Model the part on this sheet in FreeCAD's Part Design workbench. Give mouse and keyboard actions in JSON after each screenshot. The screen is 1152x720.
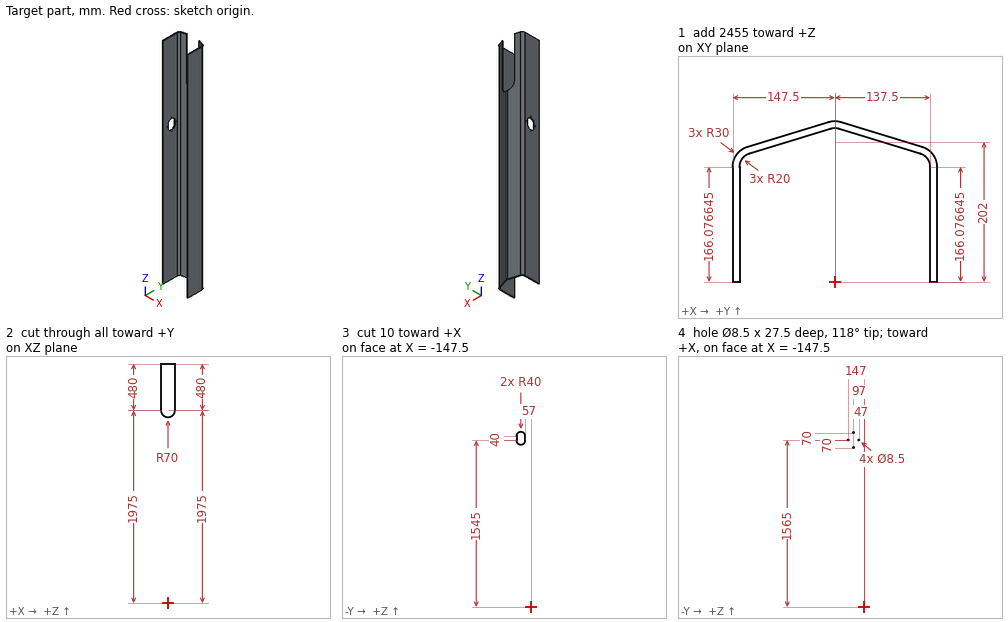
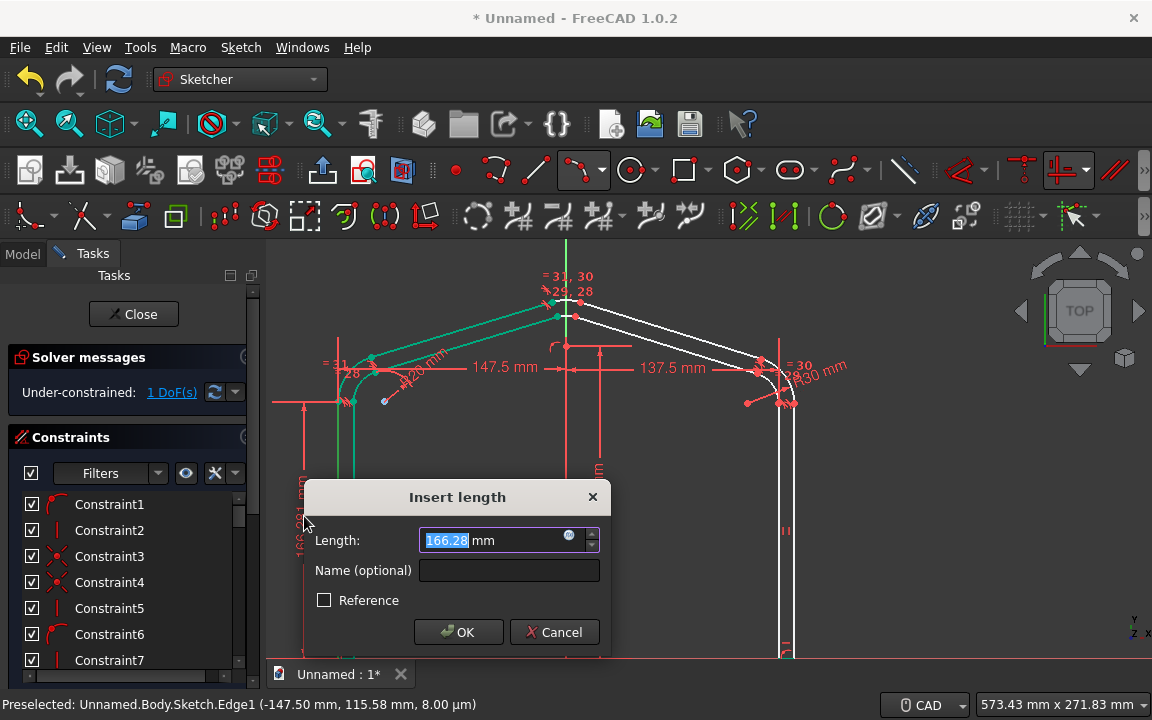
{"action": "type", "text": "166.076645"}
{"action": "key", "text": "Return"}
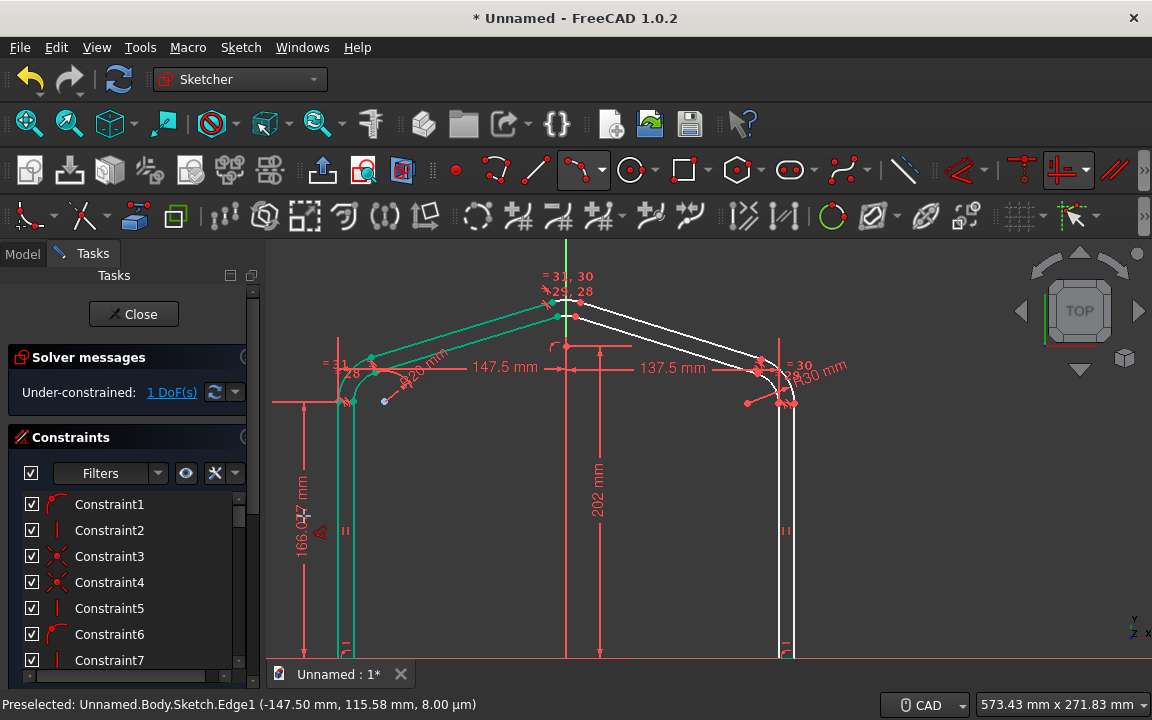
{"action": "left_click", "coordinate": [779, 480]}
{"action": "left_click", "coordinate": [813, 517]}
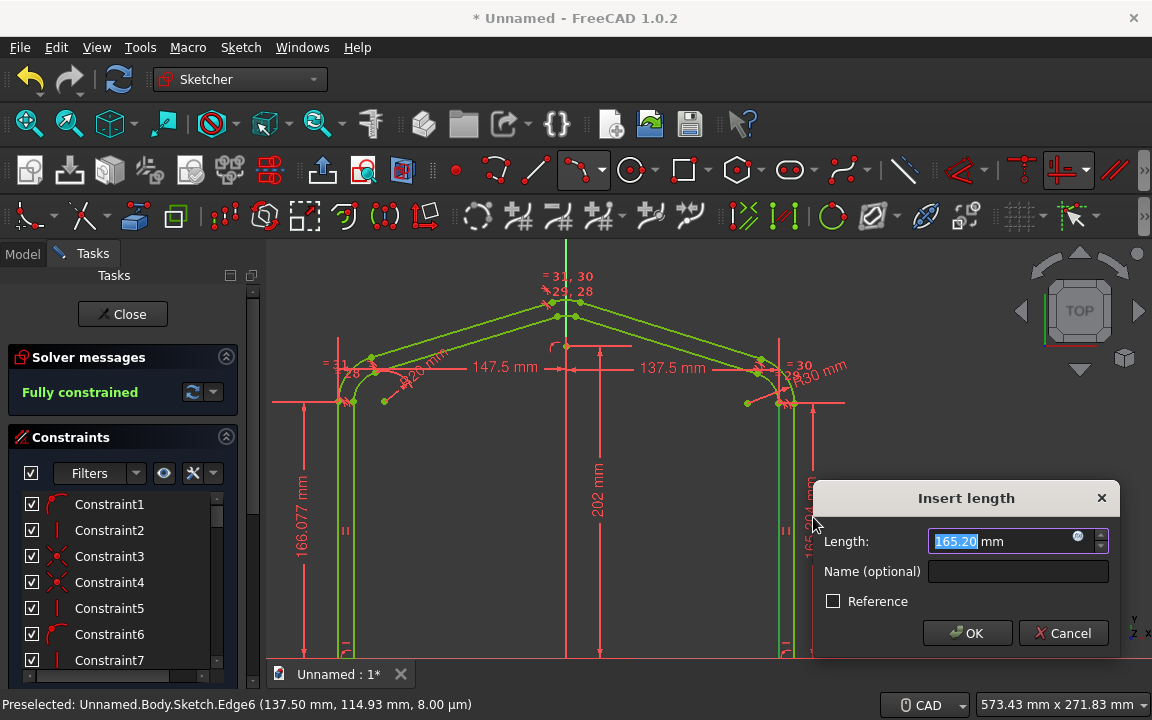
{"action": "type", "text": "166.076645"}
{"action": "key", "text": "Return"}
{"action": "key", "text": "Escape"}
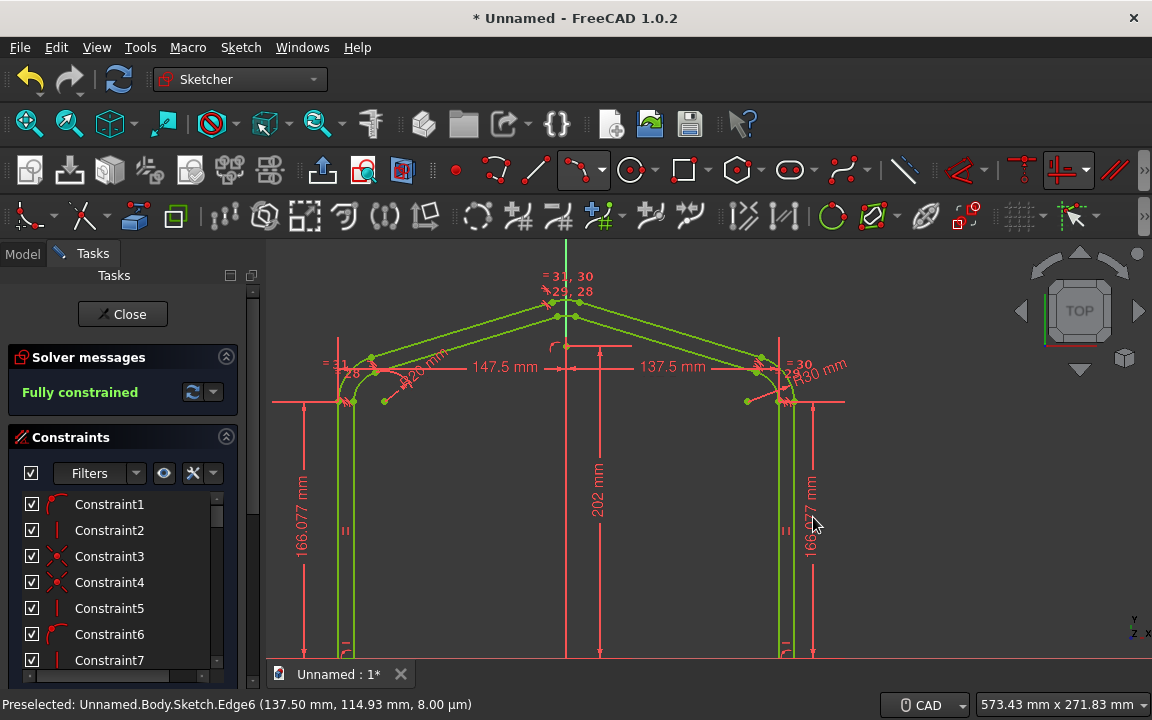
{"action": "left_click", "coordinate": [123, 314]}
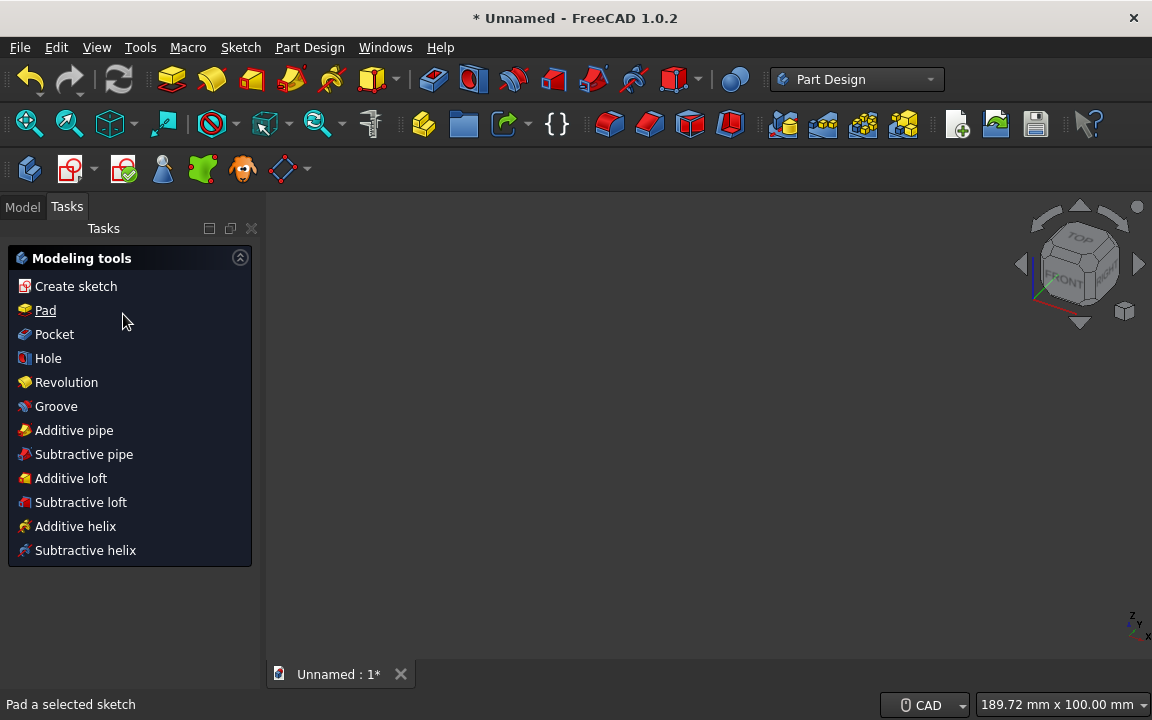
{"action": "left_click", "coordinate": [172, 80]}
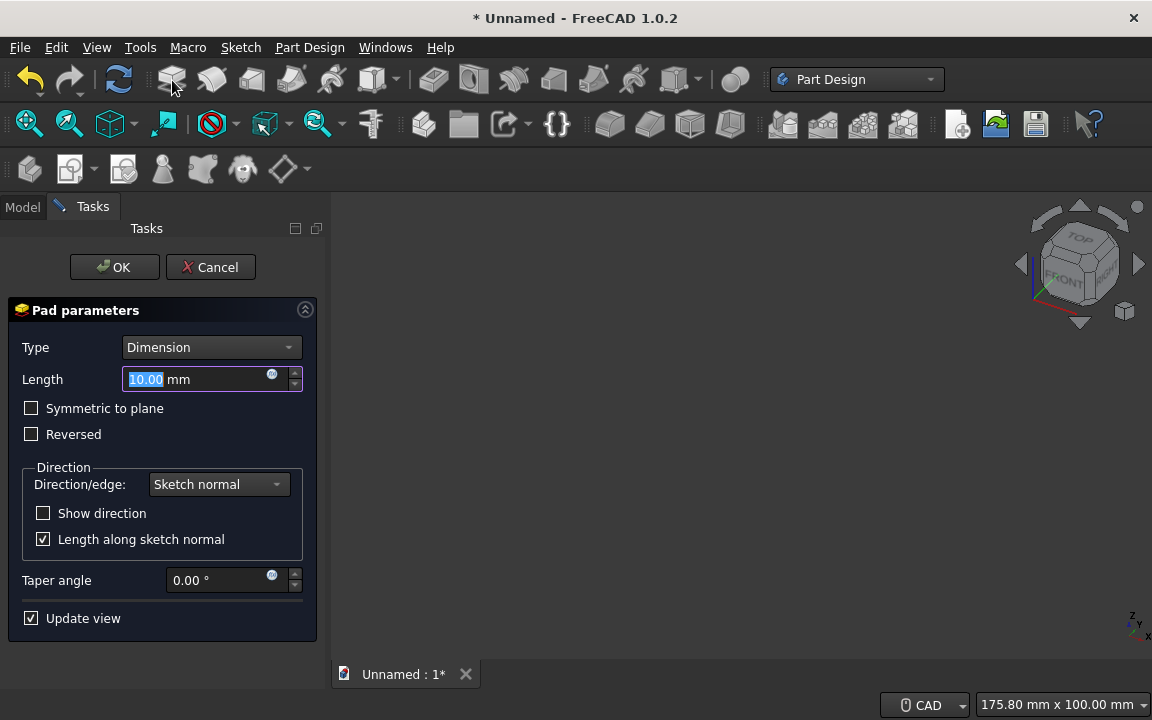
{"action": "type", "text": "2455"}
{"action": "key", "text": "Tab"}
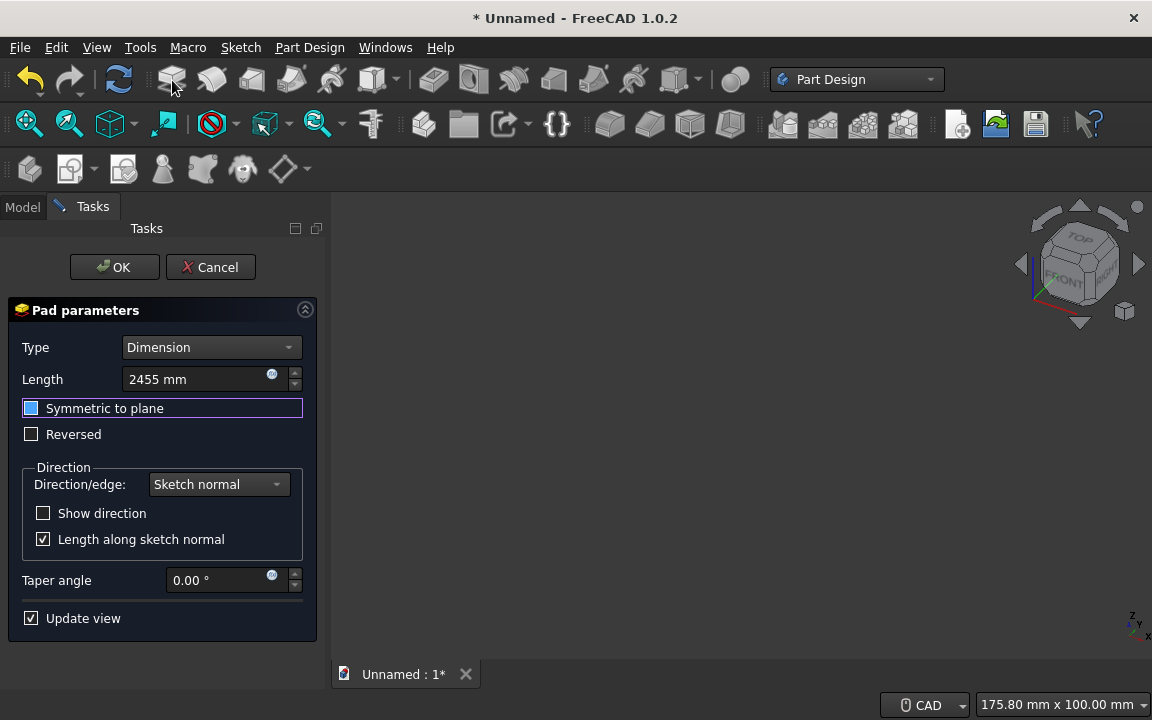
{"action": "left_click", "coordinate": [115, 267]}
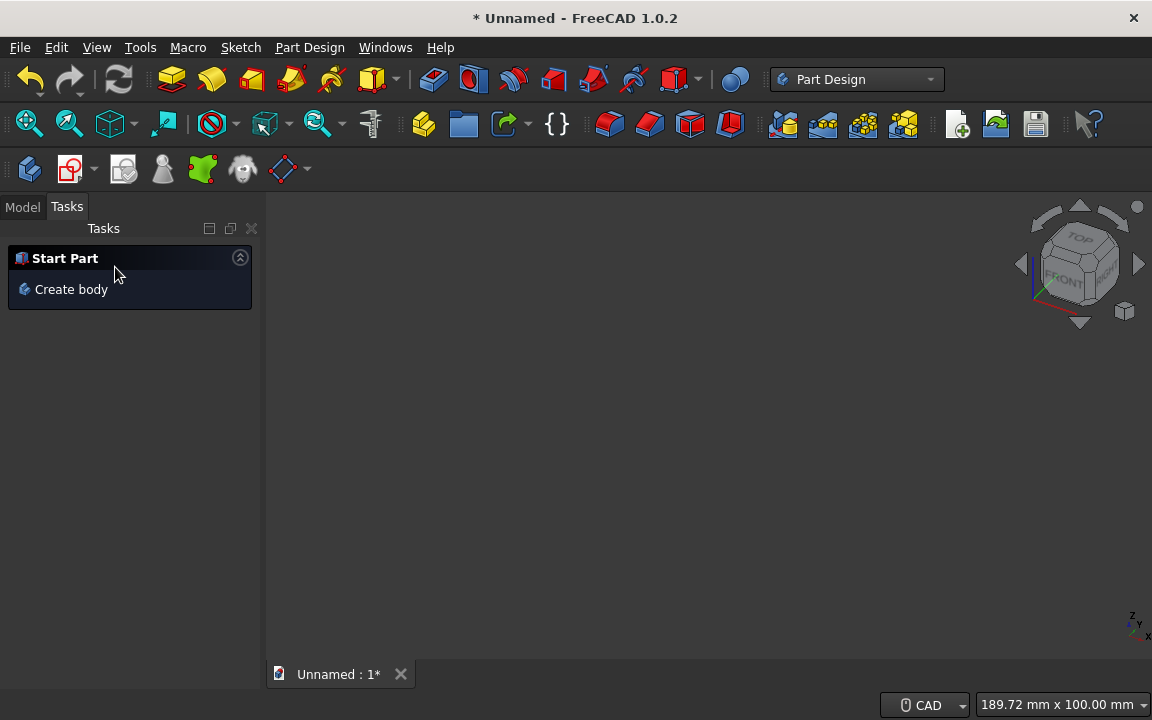
{"action": "left_click", "coordinate": [30, 124]}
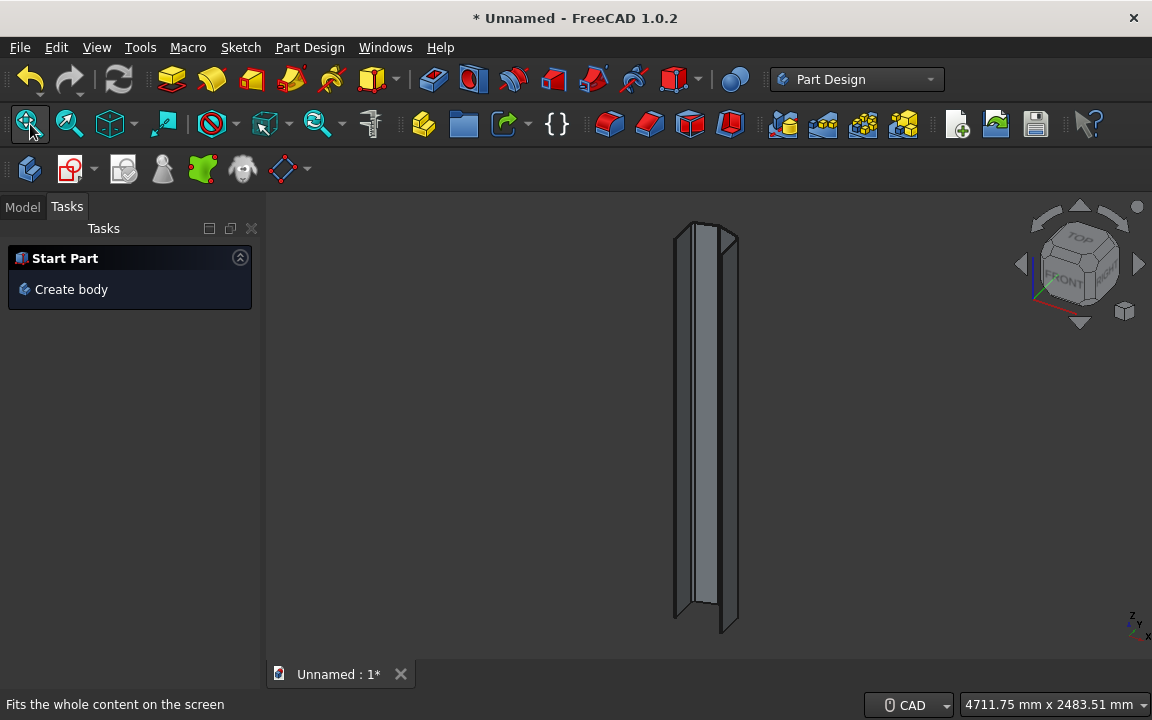
{"action": "left_click", "coordinate": [70, 170]}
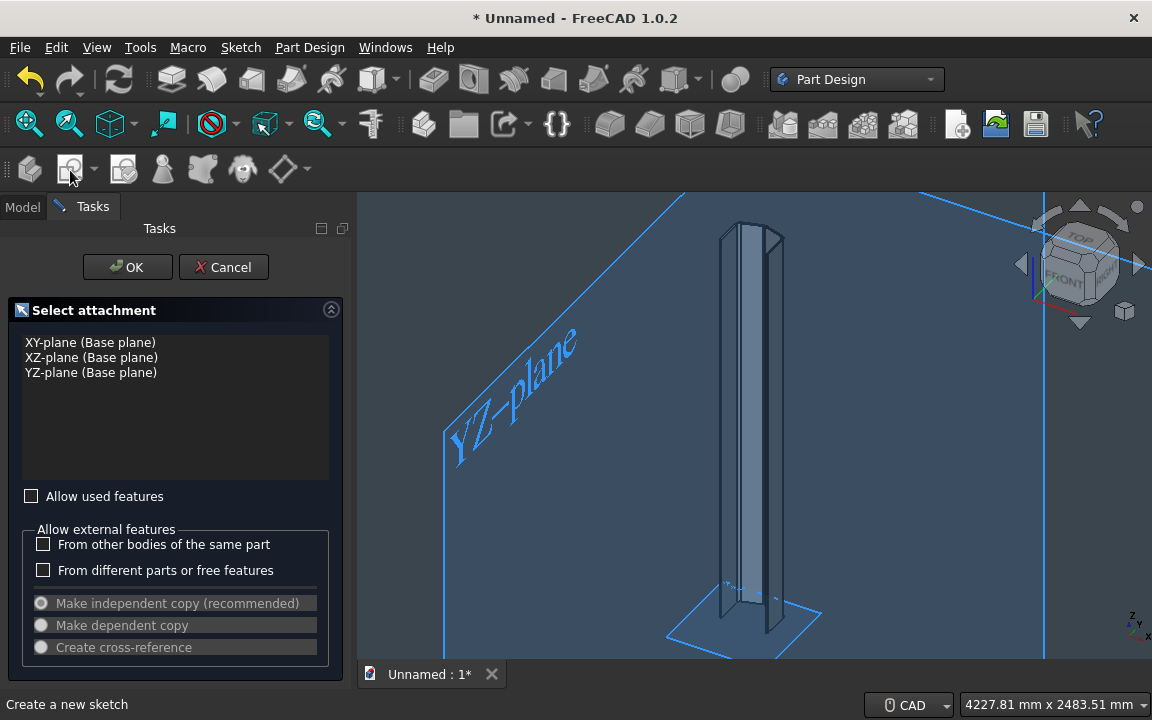
{"action": "left_click", "coordinate": [82, 358]}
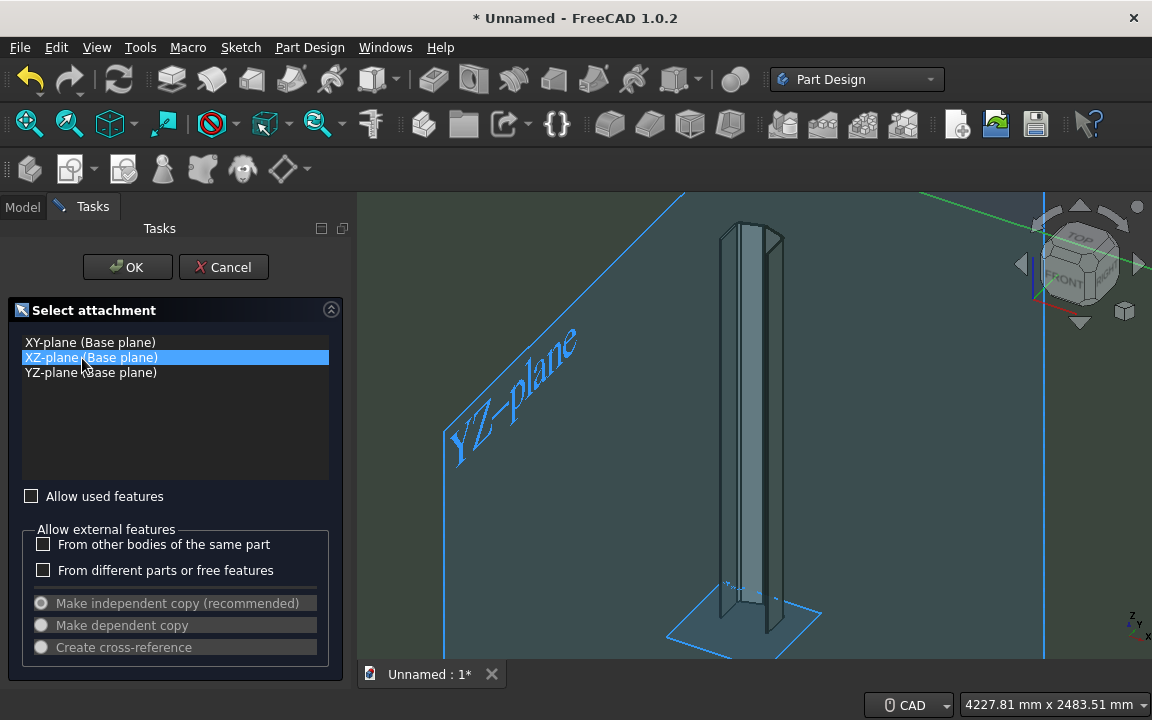
{"action": "left_click", "coordinate": [128, 267]}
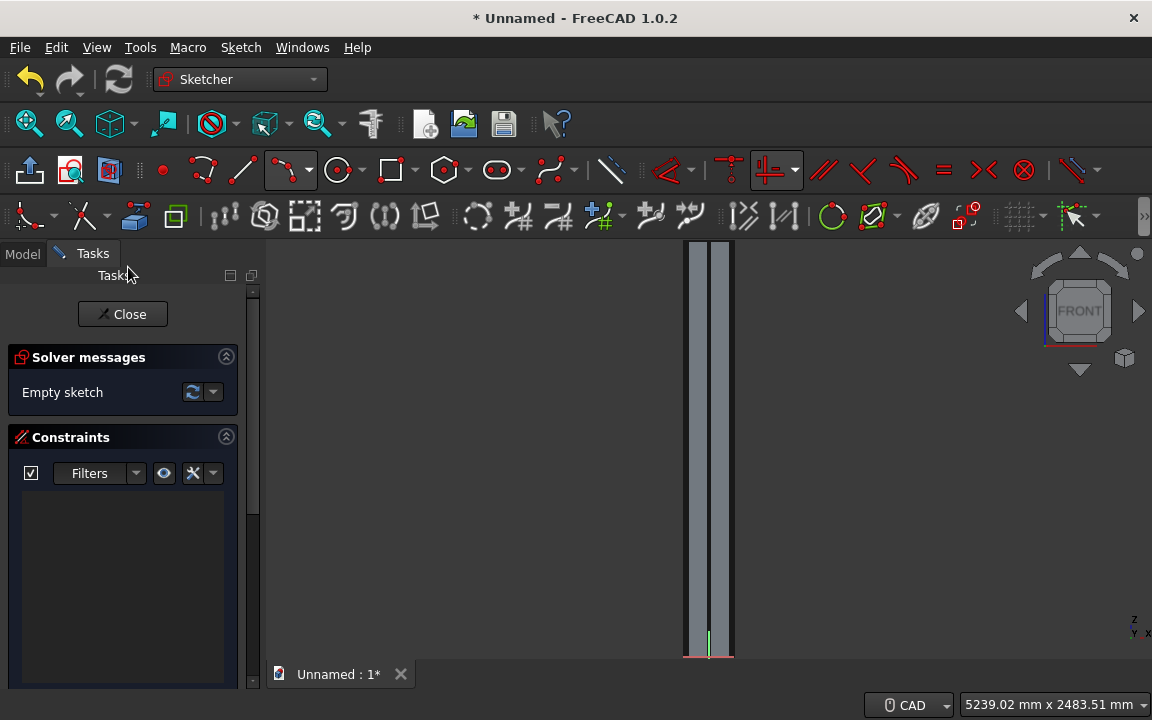
{"action": "scroll", "coordinate": [640, 449], "scroll_direction": "down", "scroll_amount": 5}